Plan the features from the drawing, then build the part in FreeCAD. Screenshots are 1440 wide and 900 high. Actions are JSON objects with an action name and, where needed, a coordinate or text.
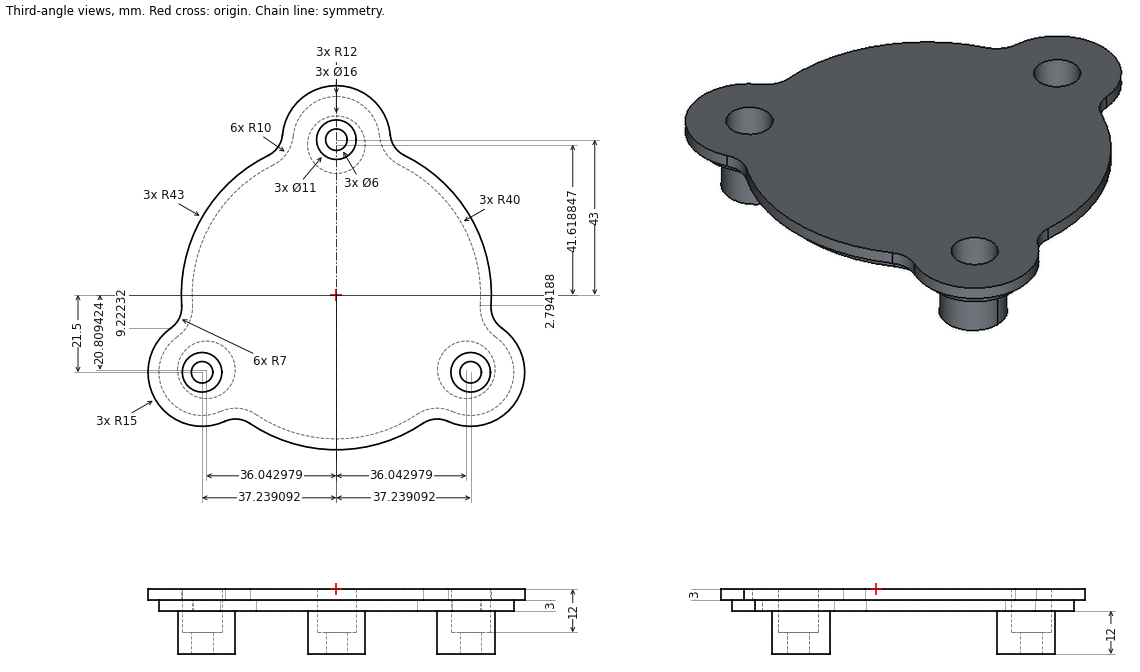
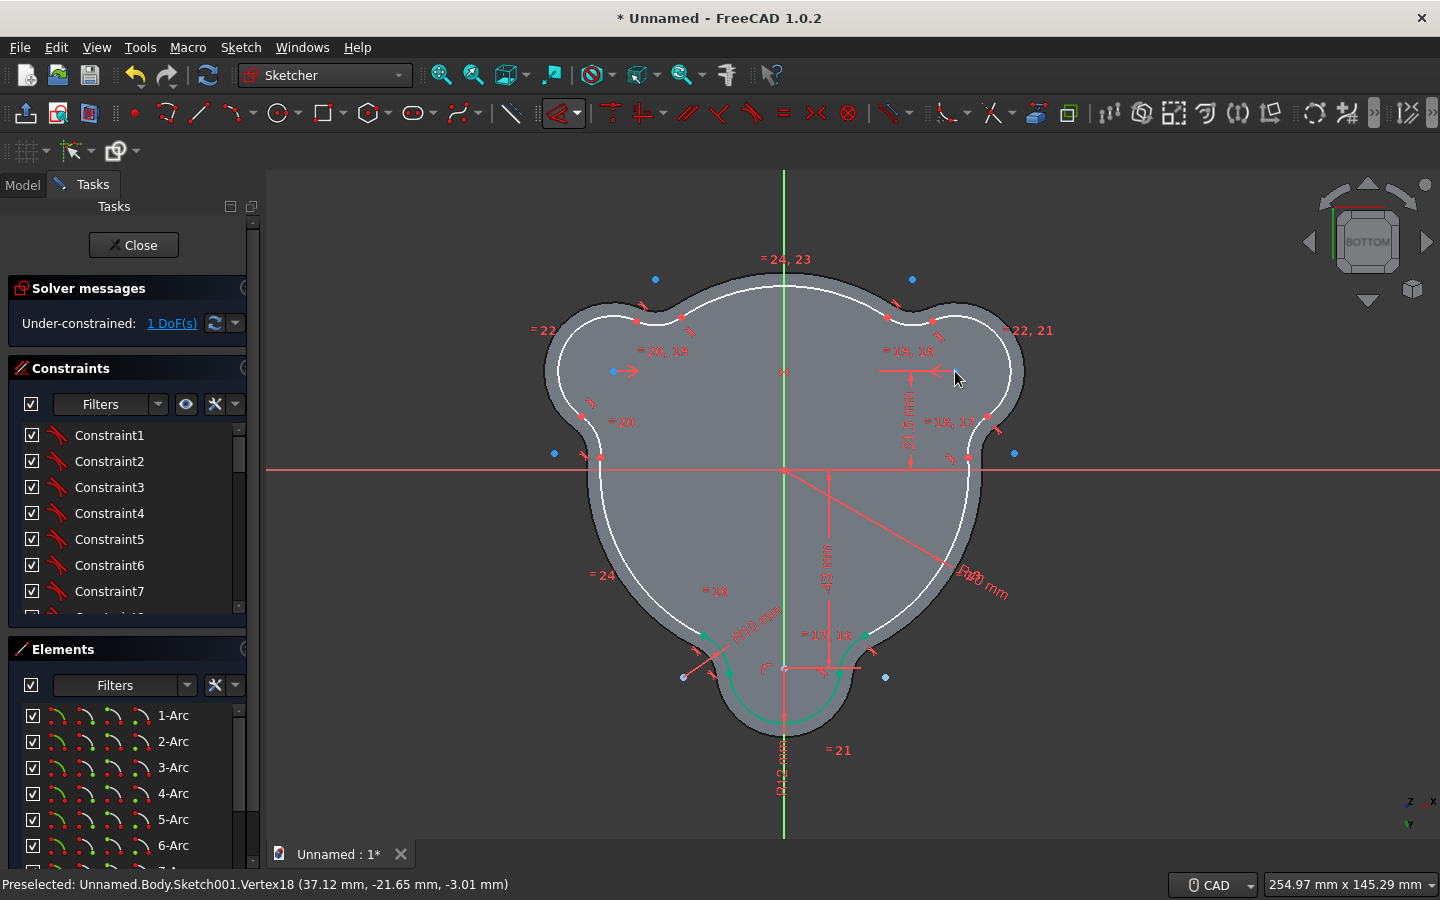
{"action": "scroll", "coordinate": [968, 457], "scroll_direction": "up", "scroll_amount": 6}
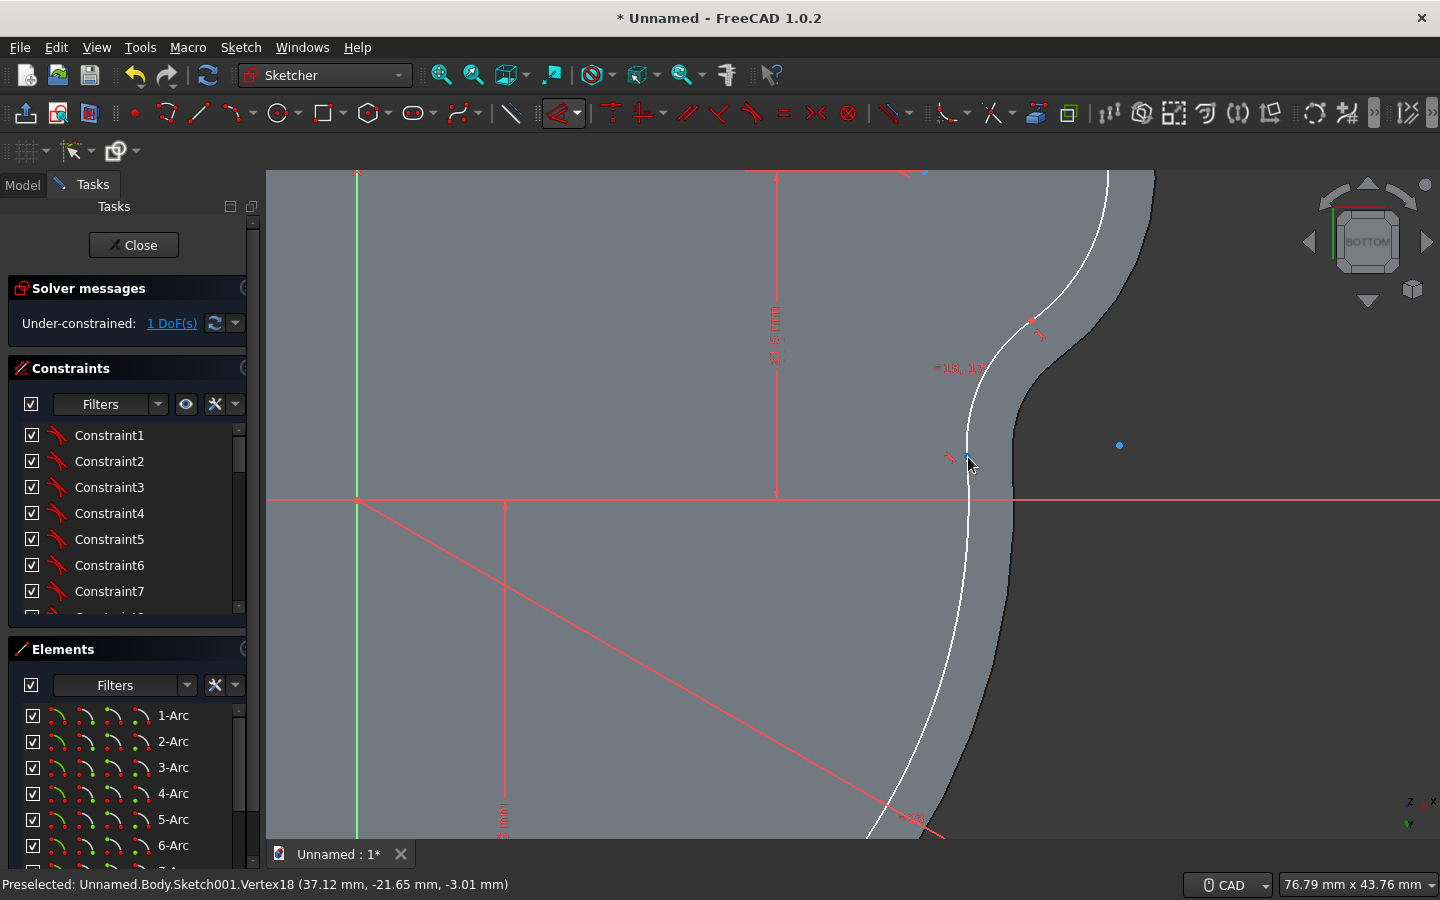
{"action": "left_click", "coordinate": [967, 456]}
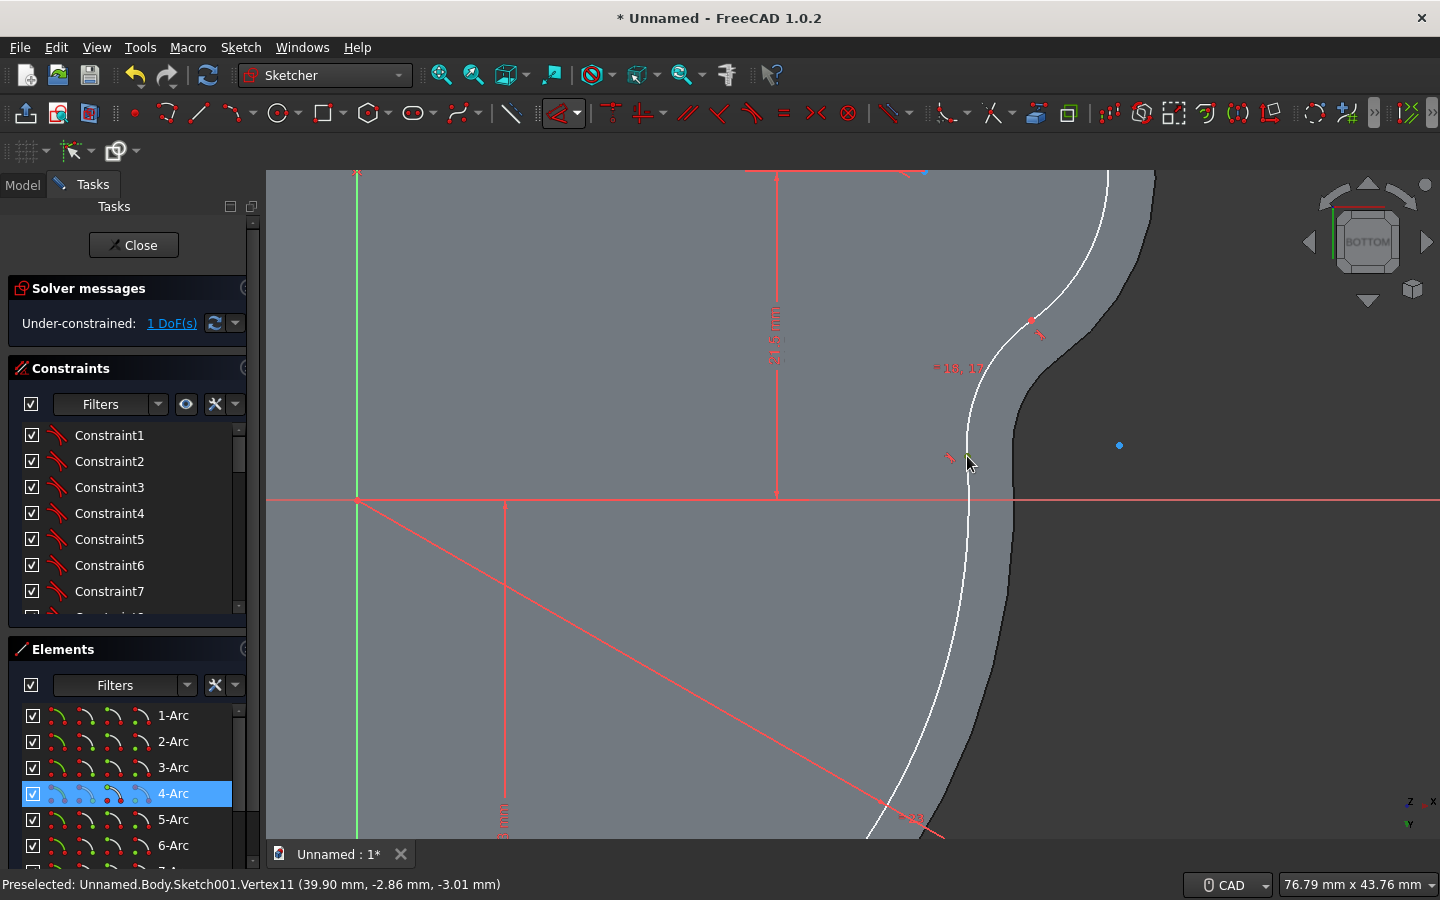
{"action": "key", "text": "i"}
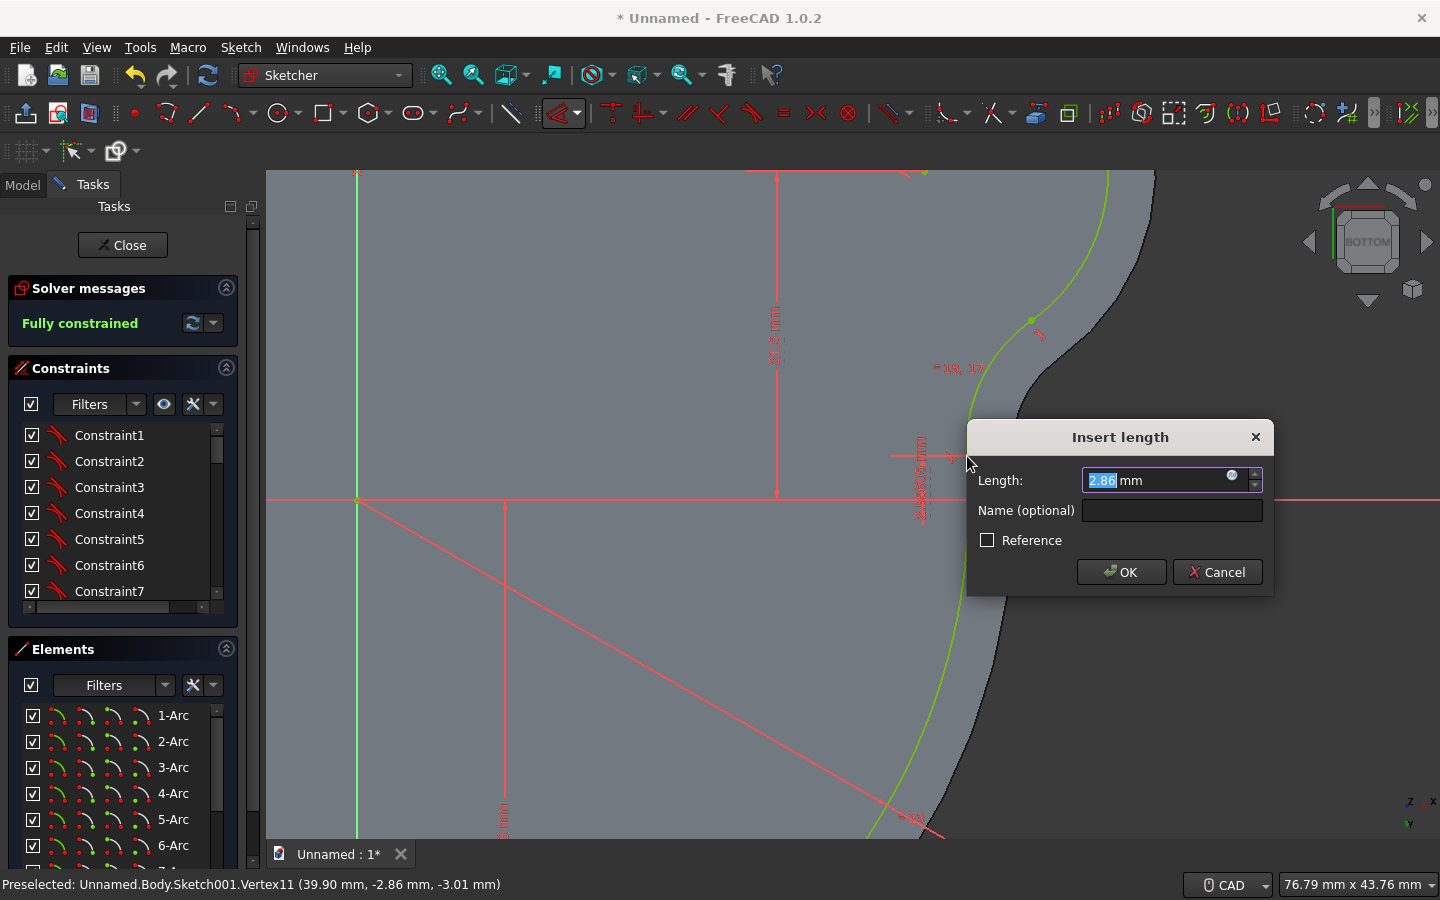
{"action": "type", "text": "2.794188"}
{"action": "key", "text": "Return"}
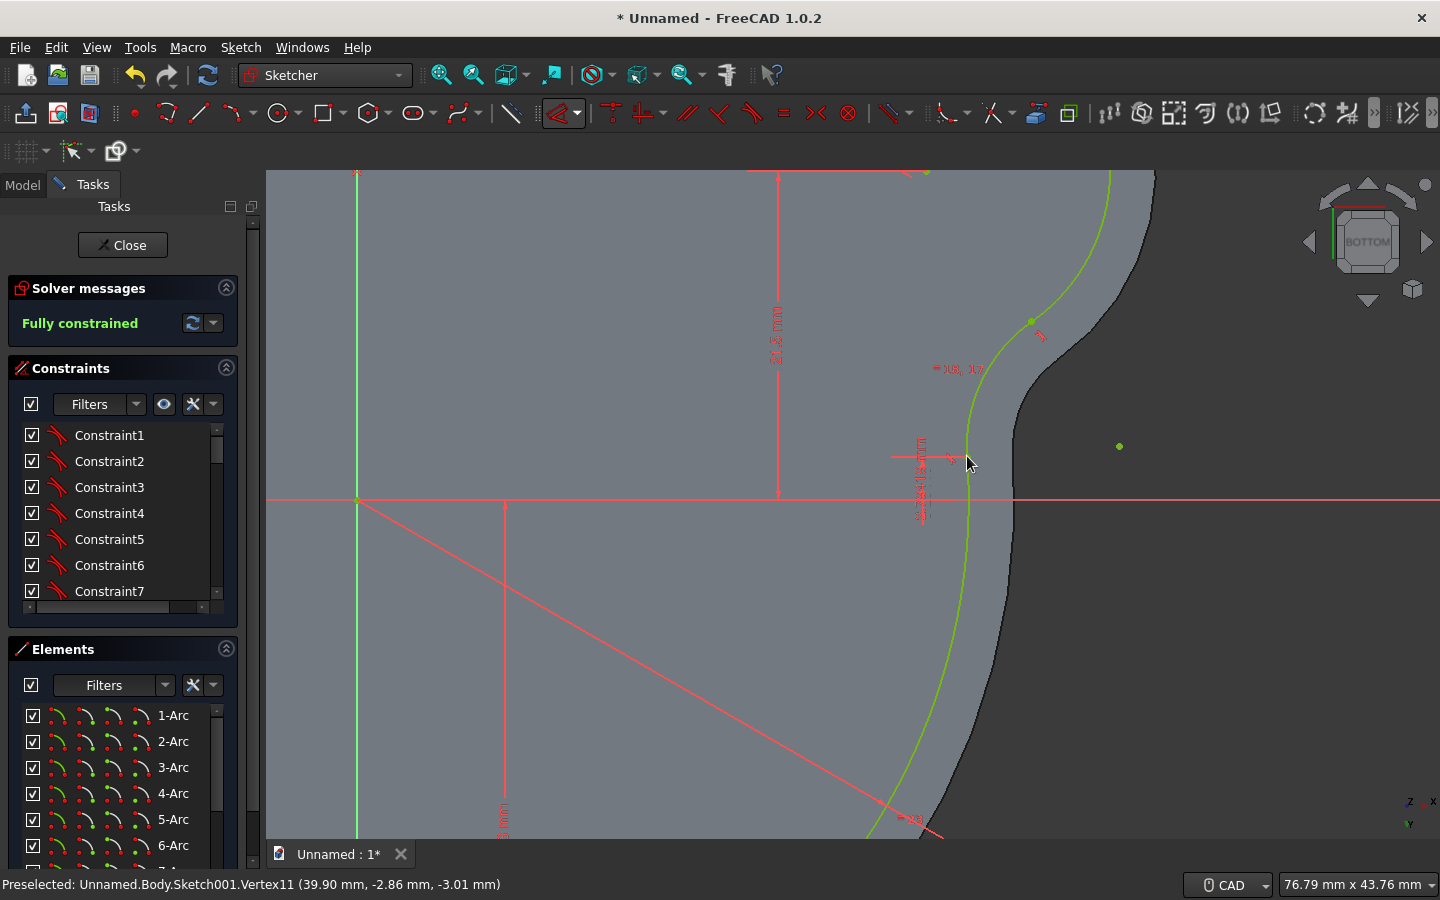
{"action": "left_click", "coordinate": [123, 245]}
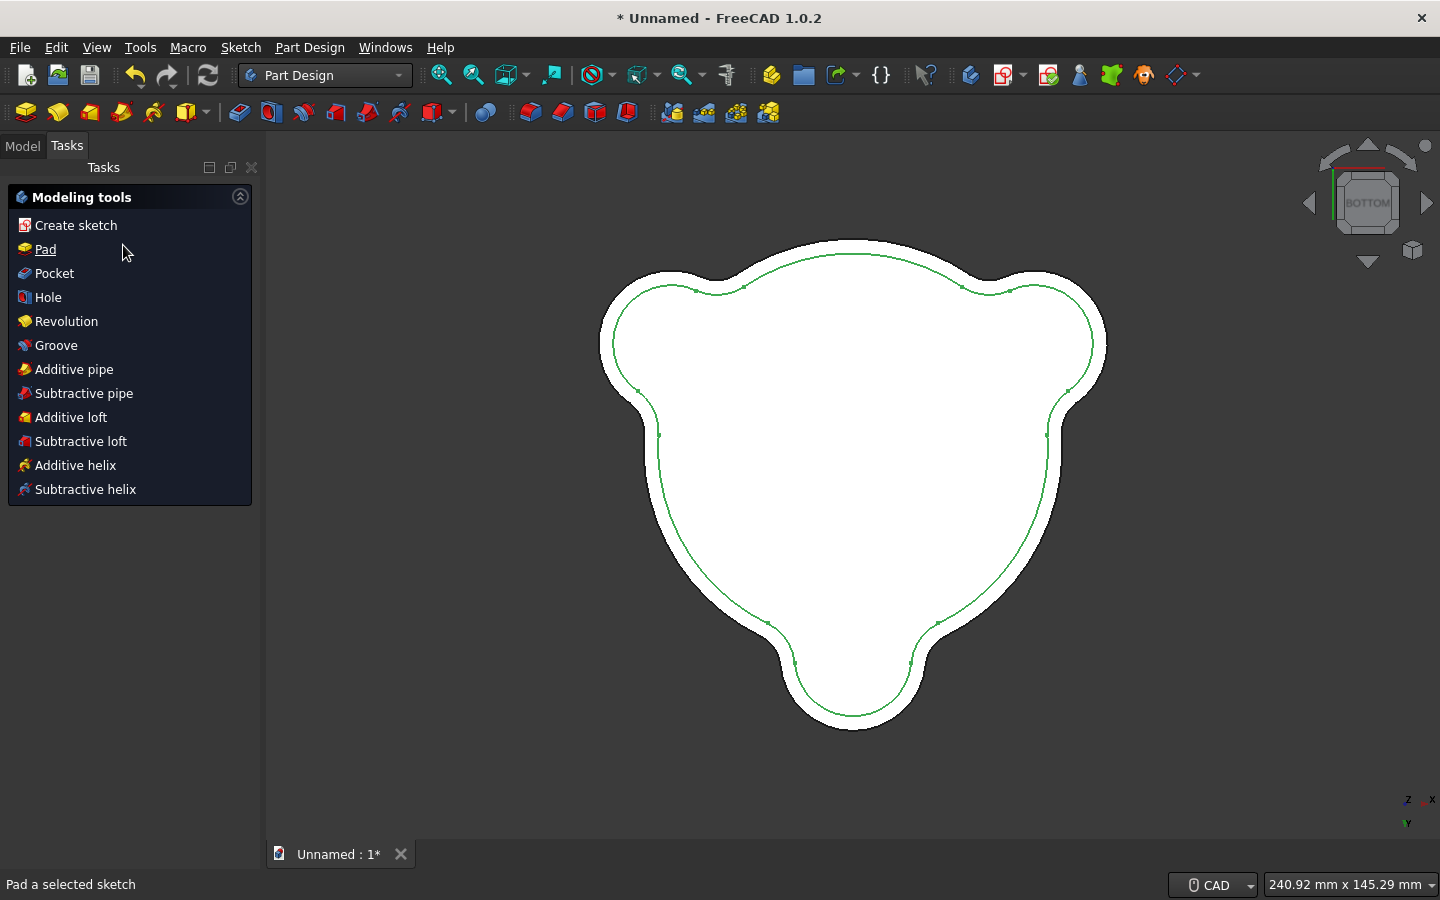
{"action": "left_click", "coordinate": [26, 112]}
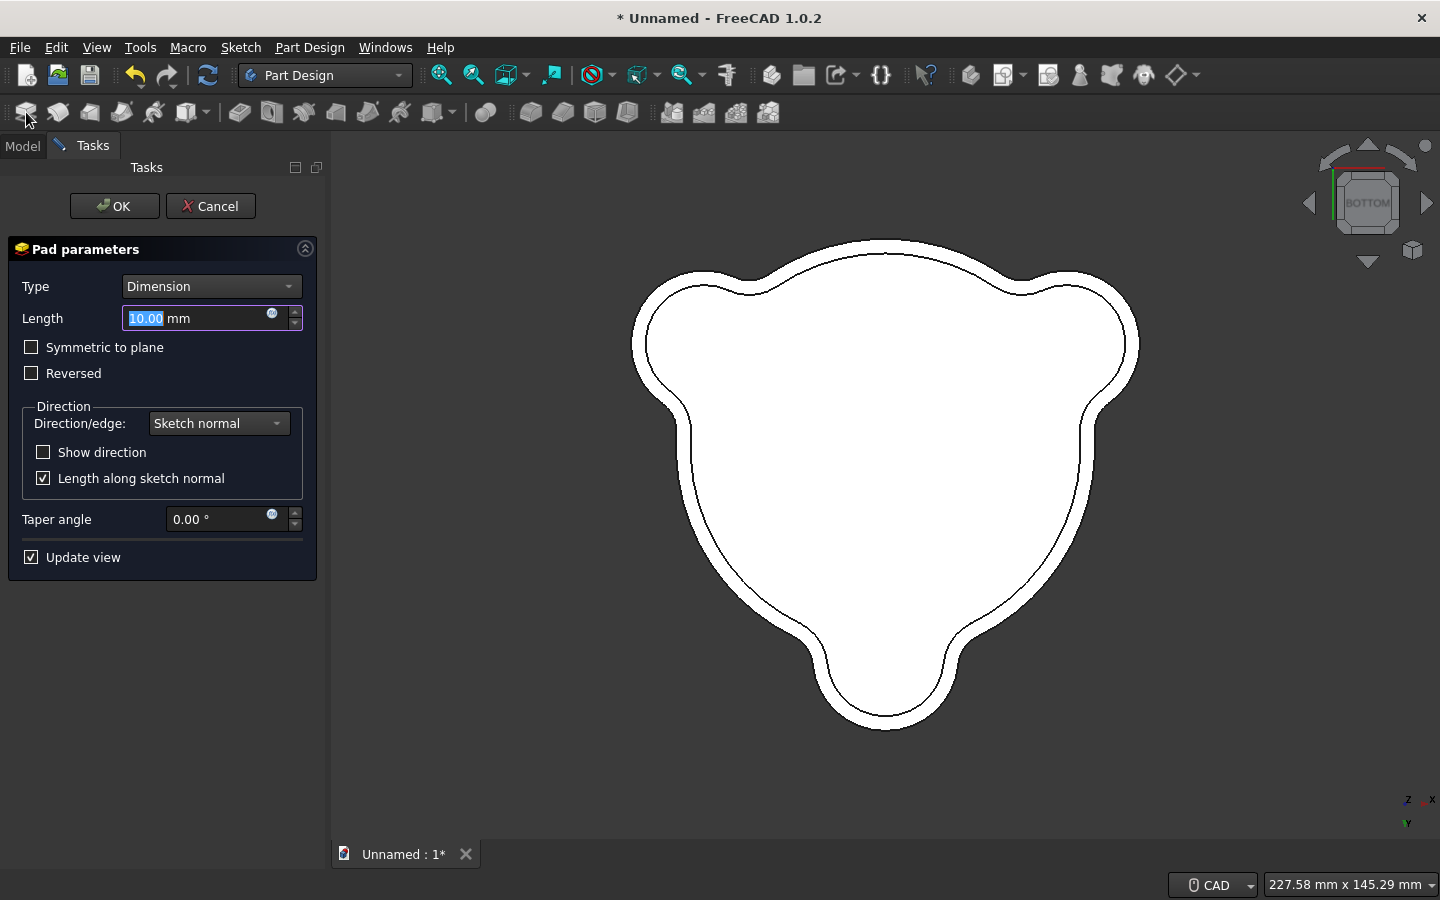
{"action": "type", "text": "3"}
{"action": "key", "text": "Tab"}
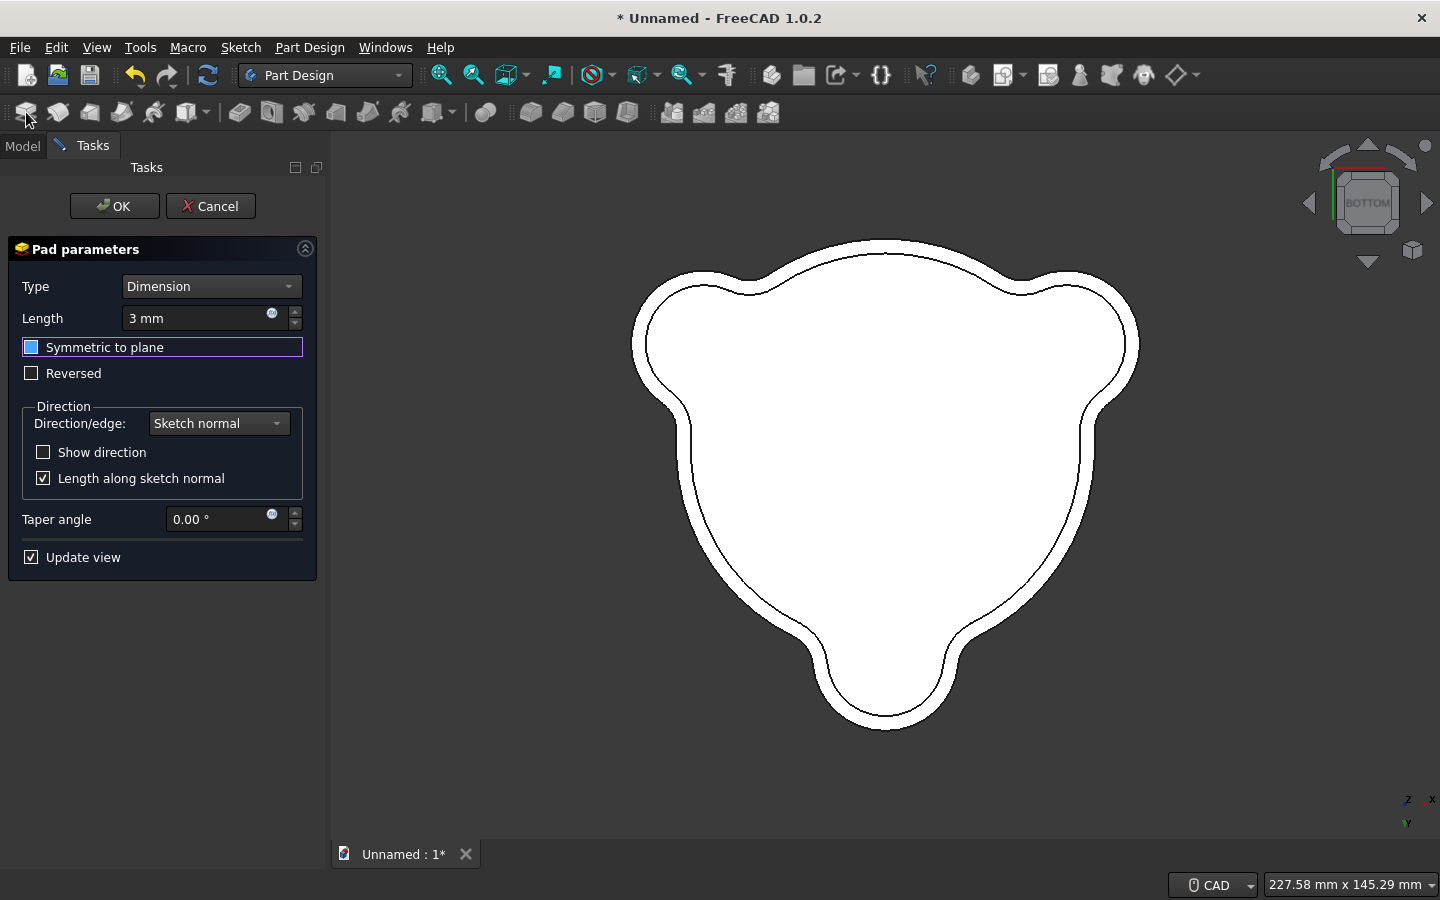
{"action": "left_click", "coordinate": [115, 206]}